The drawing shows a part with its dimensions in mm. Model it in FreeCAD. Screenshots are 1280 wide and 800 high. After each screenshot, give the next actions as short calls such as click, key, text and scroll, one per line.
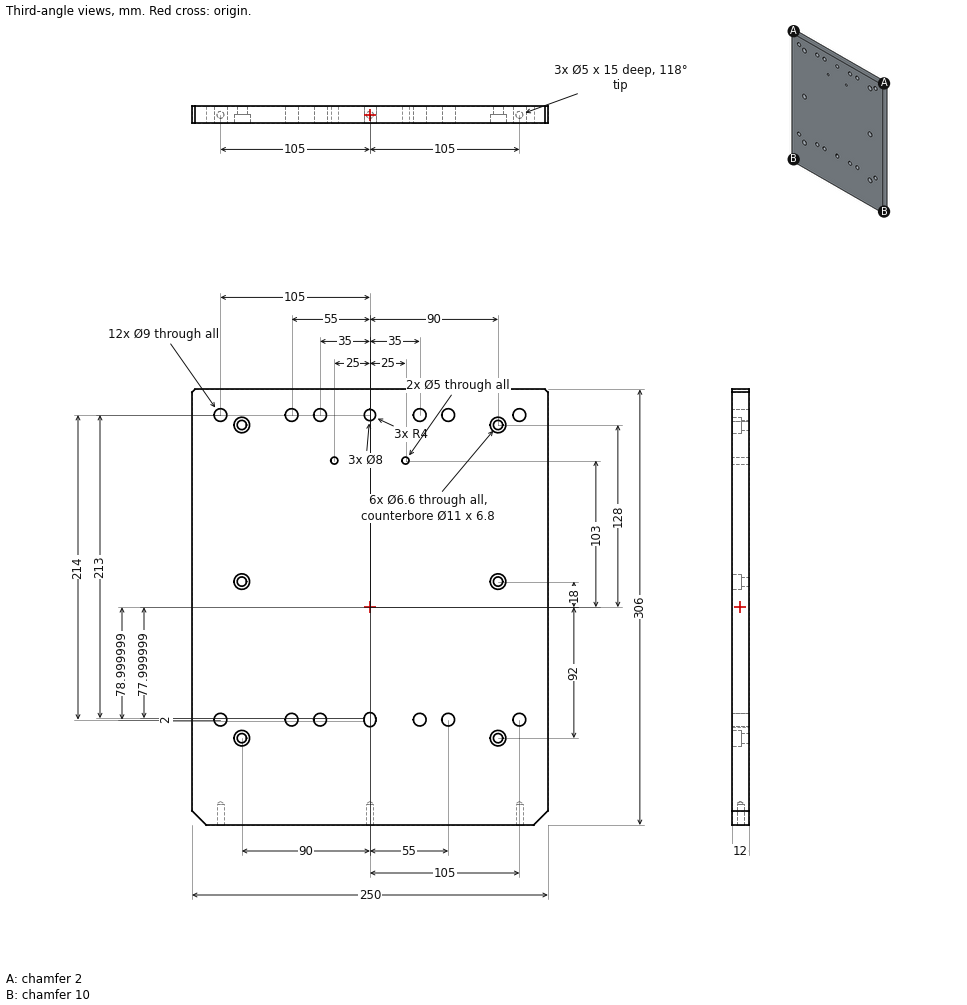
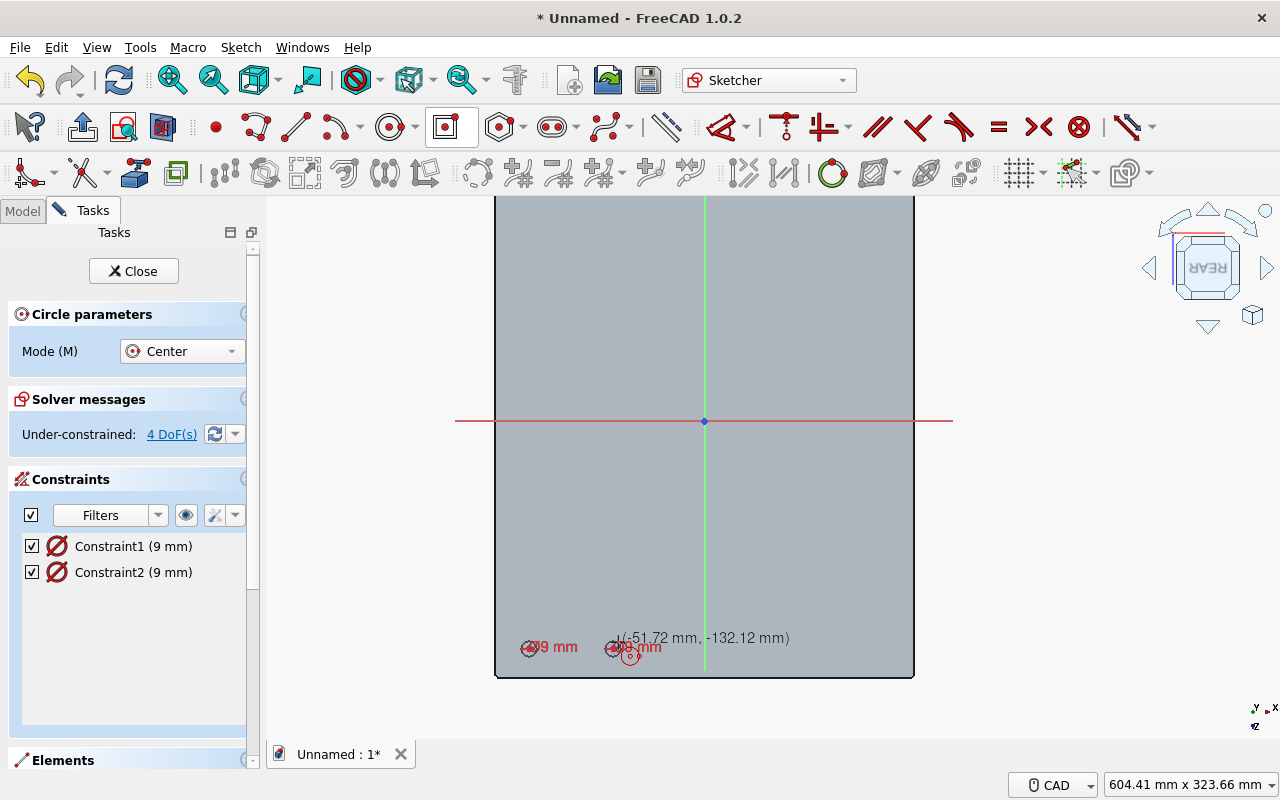
scroll(529, 289, up, 6)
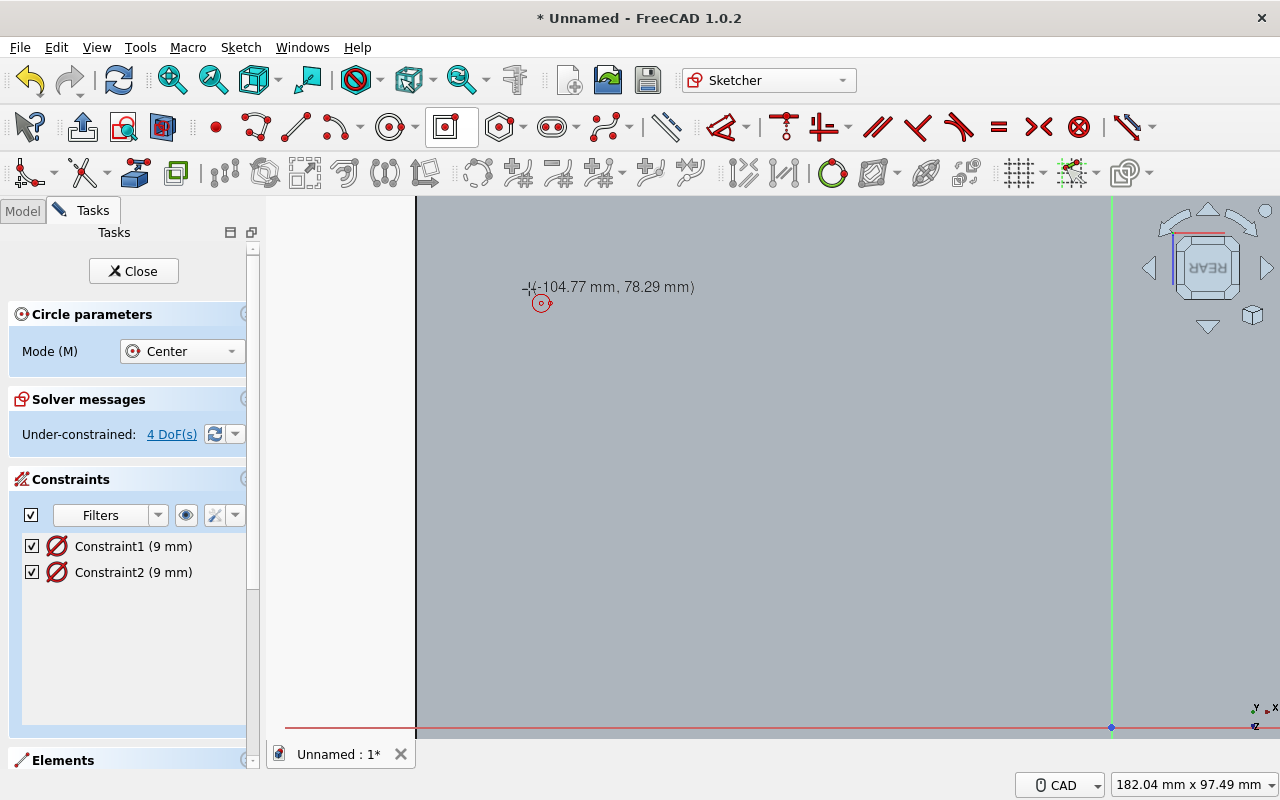
scroll(529, 288, down, 6)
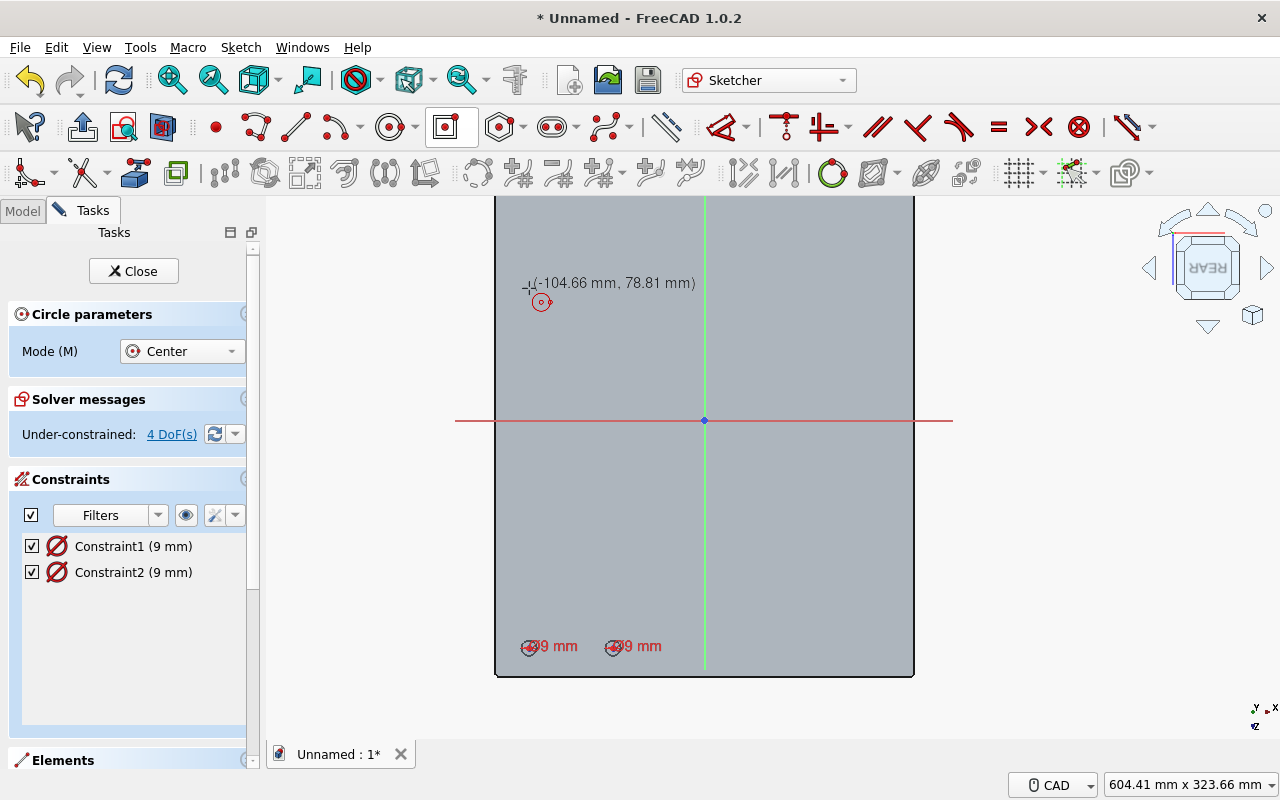
click(529, 288)
move(534, 283)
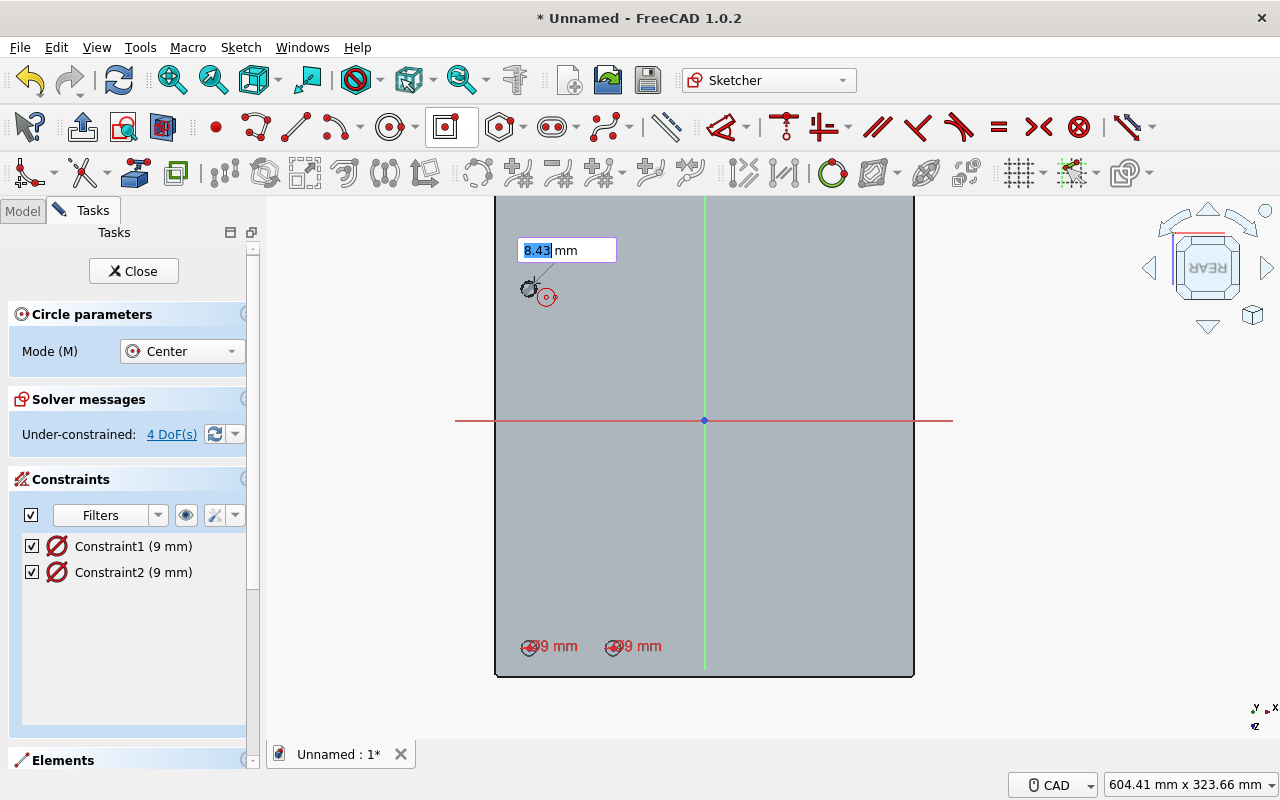
text(9)
key(Return)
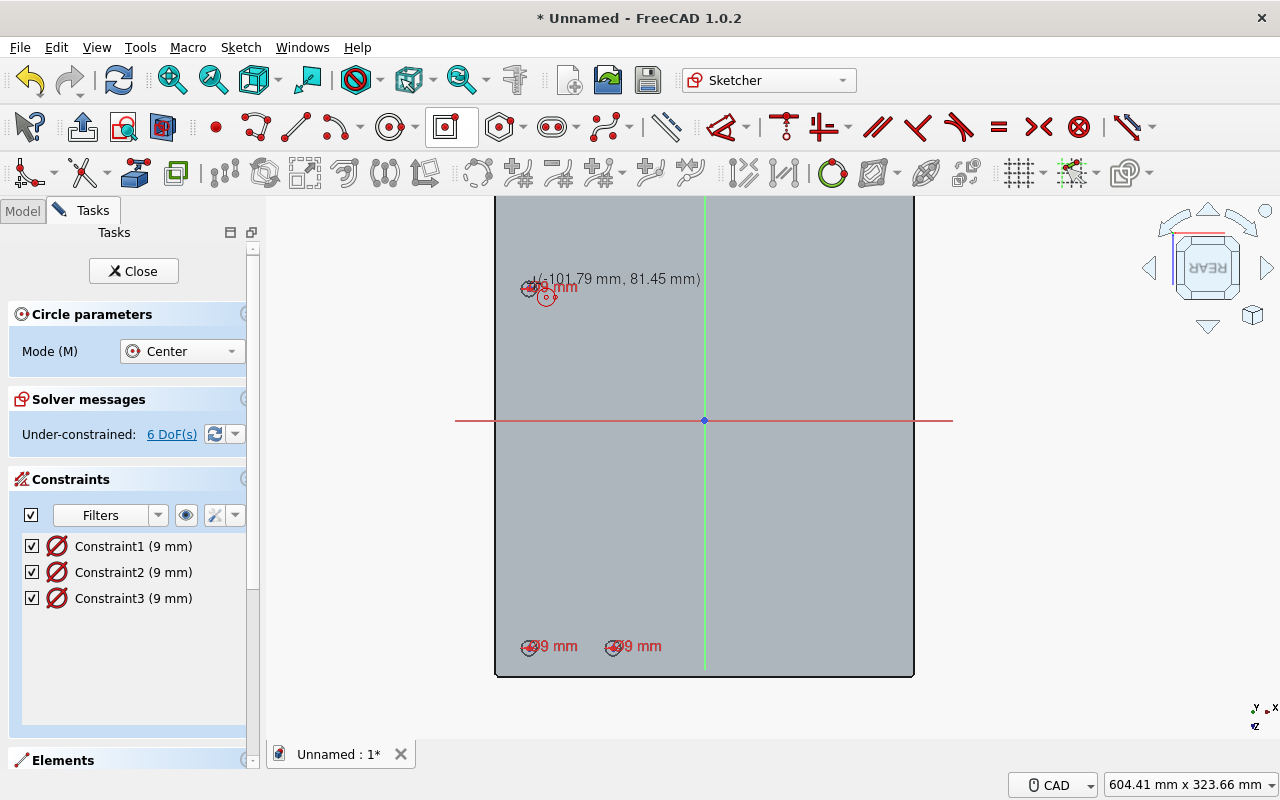
scroll(613, 288, up, 6)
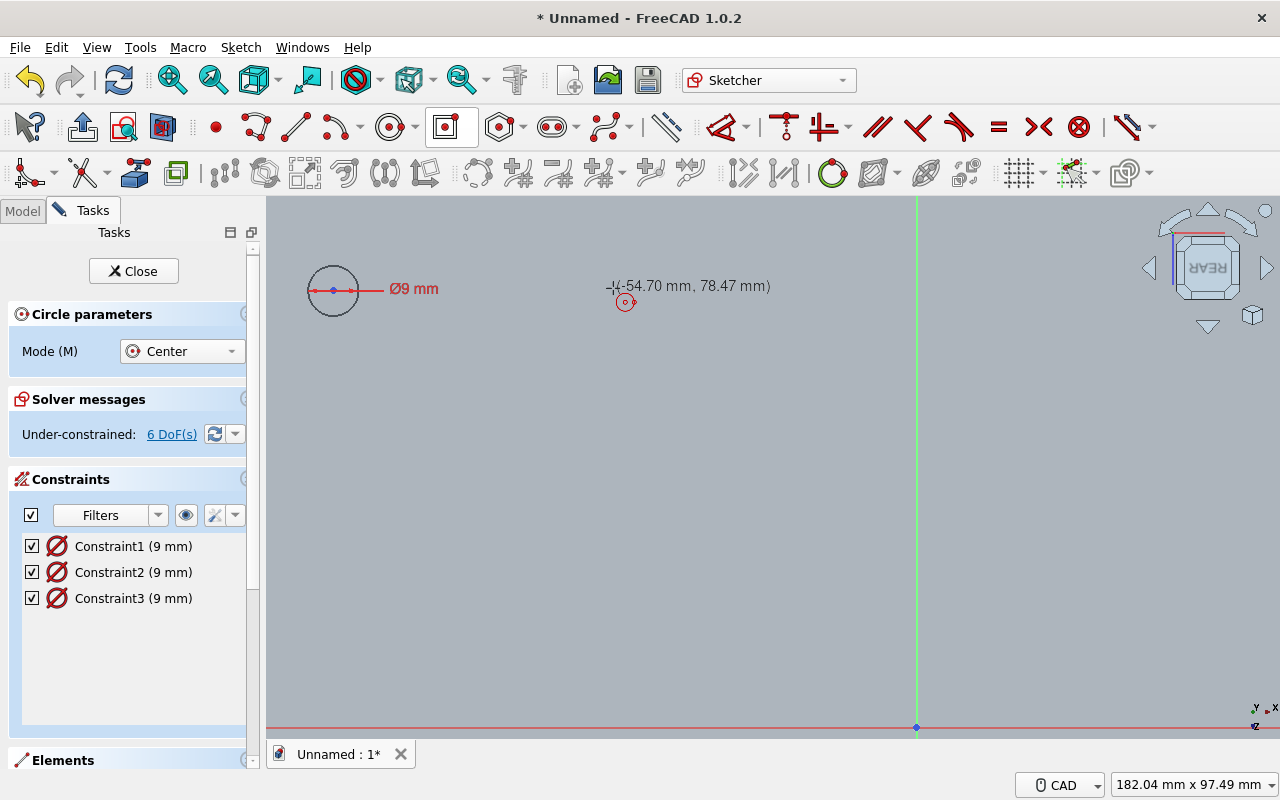
scroll(613, 288, down, 6)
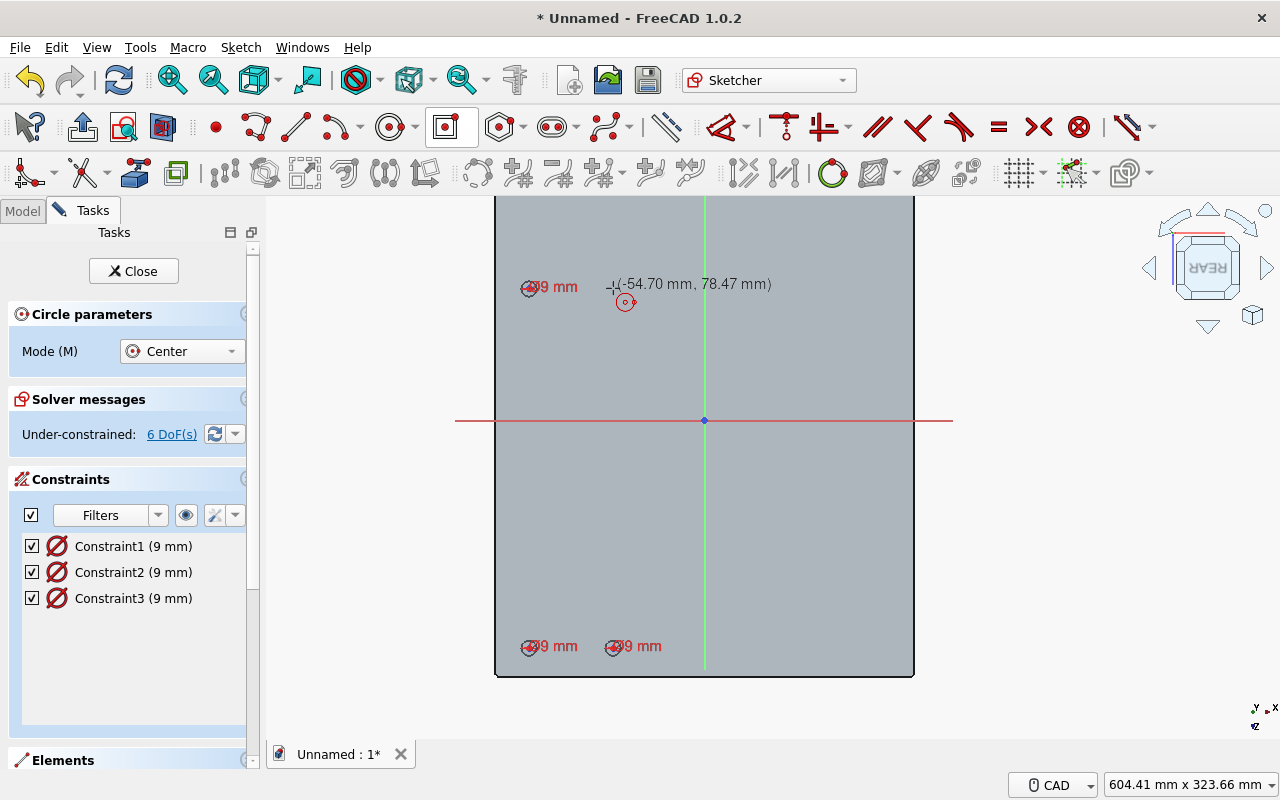
click(613, 288)
move(618, 283)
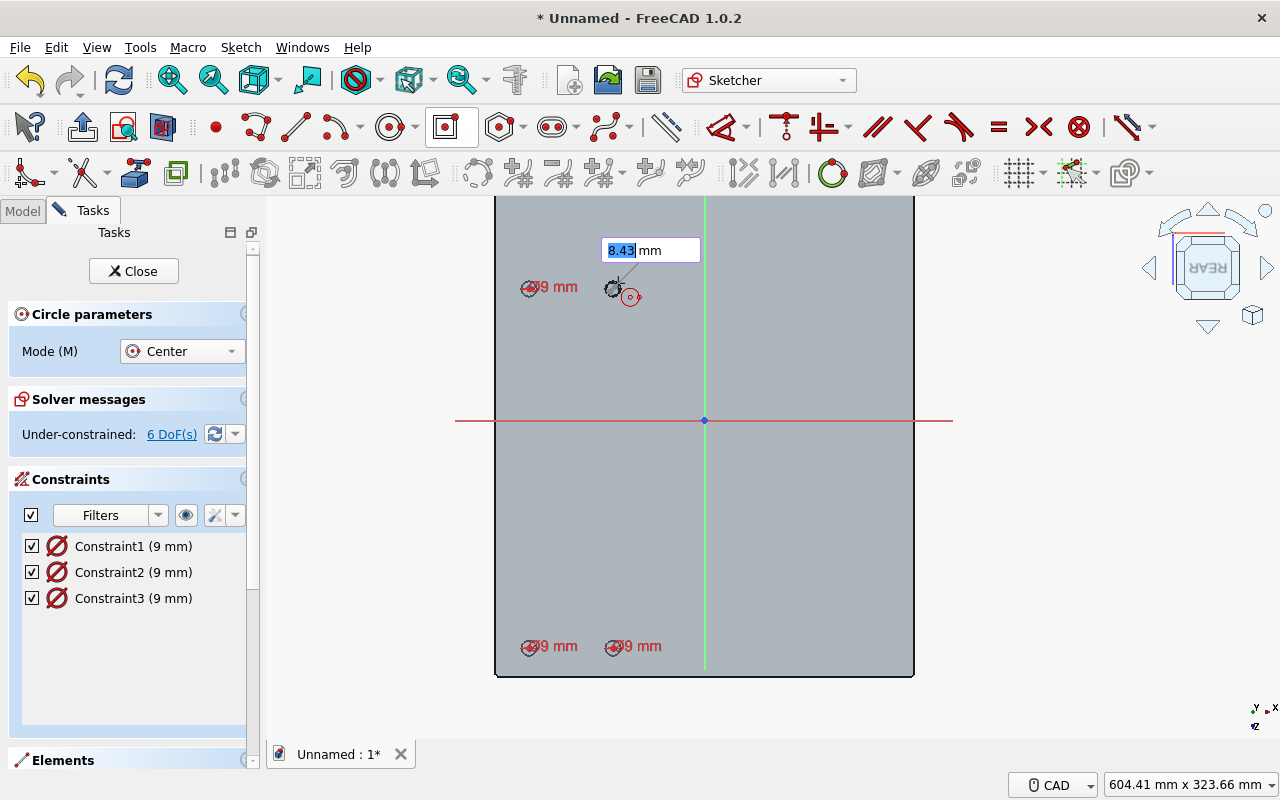
text(9)
key(Return)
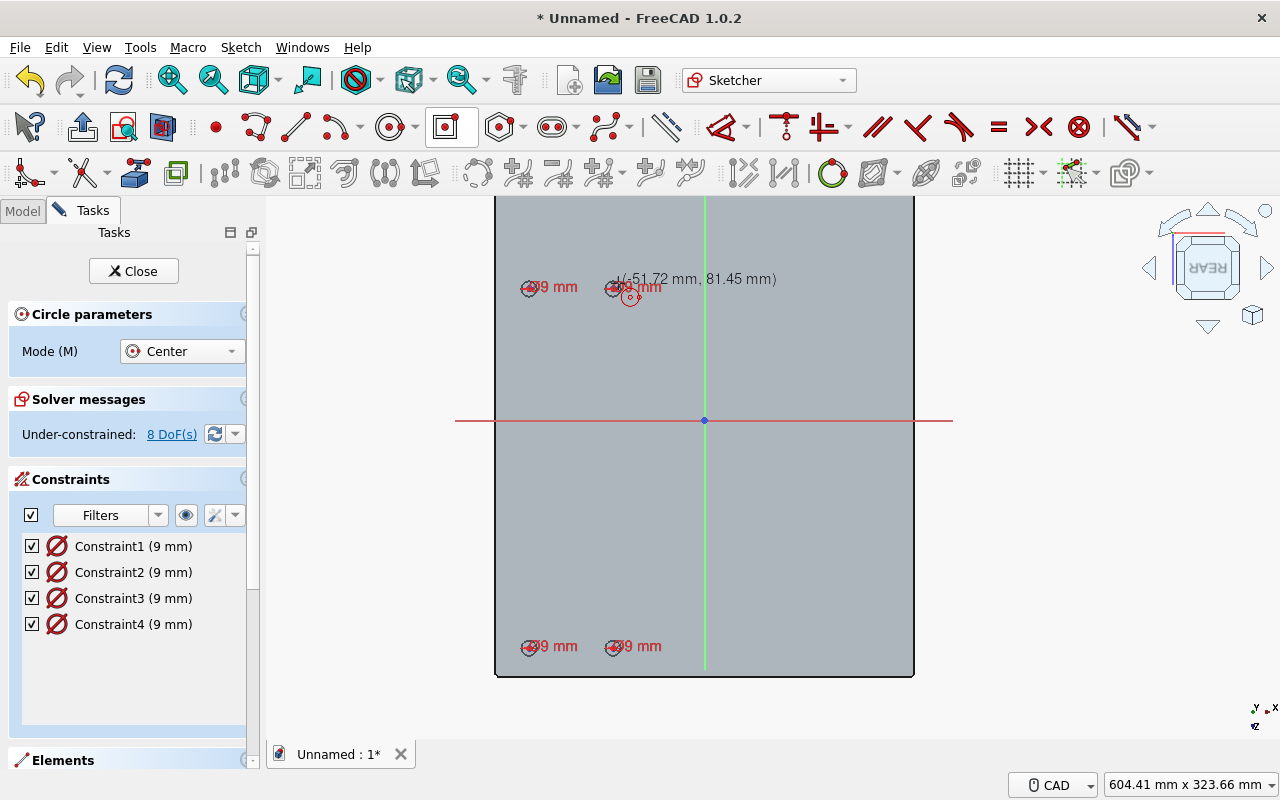
scroll(797, 288, up, 6)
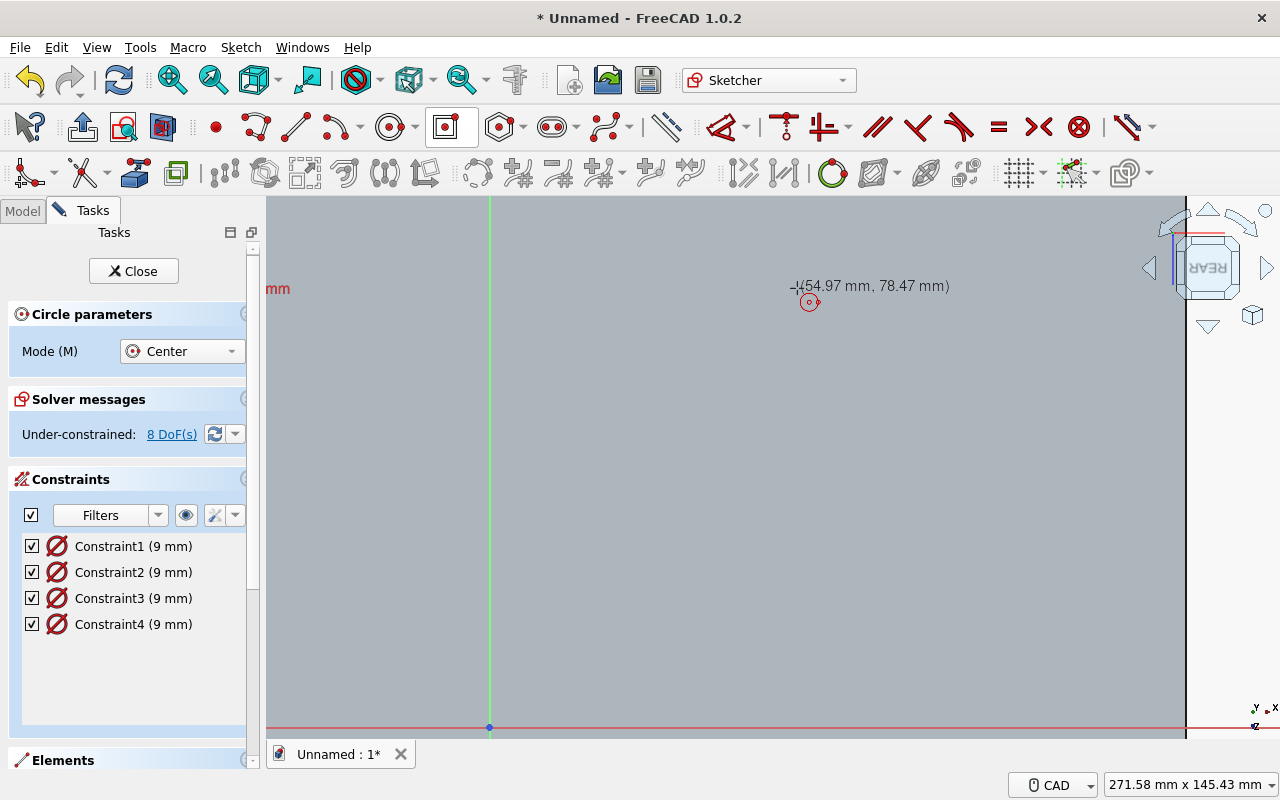
scroll(797, 288, down, 6)